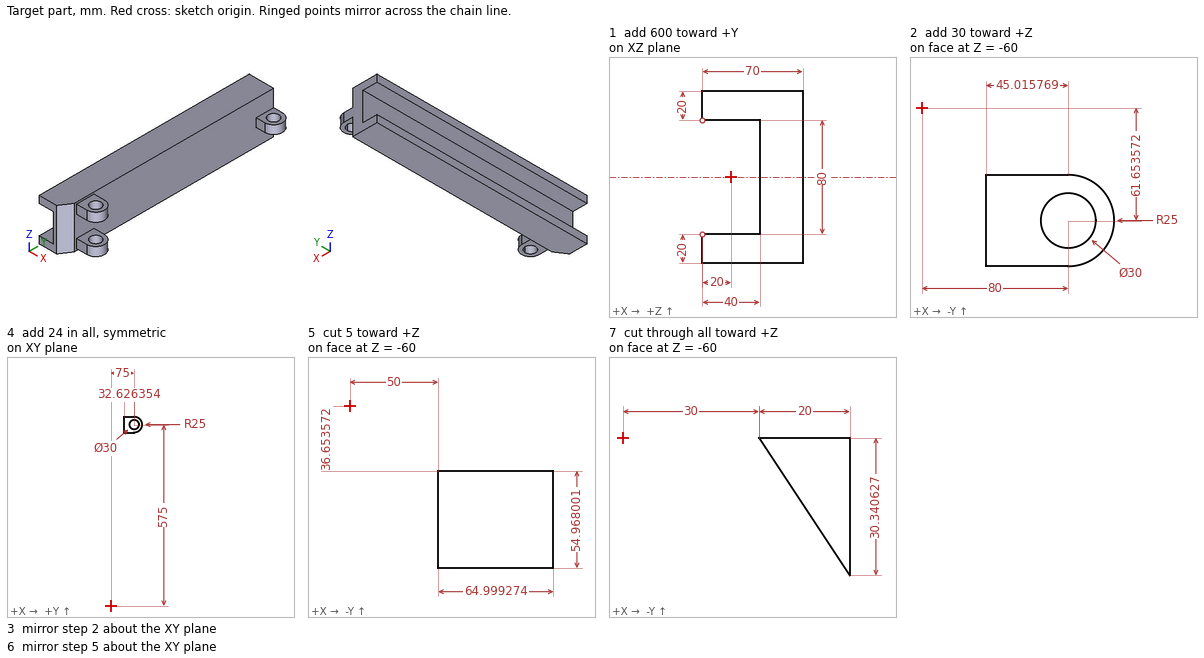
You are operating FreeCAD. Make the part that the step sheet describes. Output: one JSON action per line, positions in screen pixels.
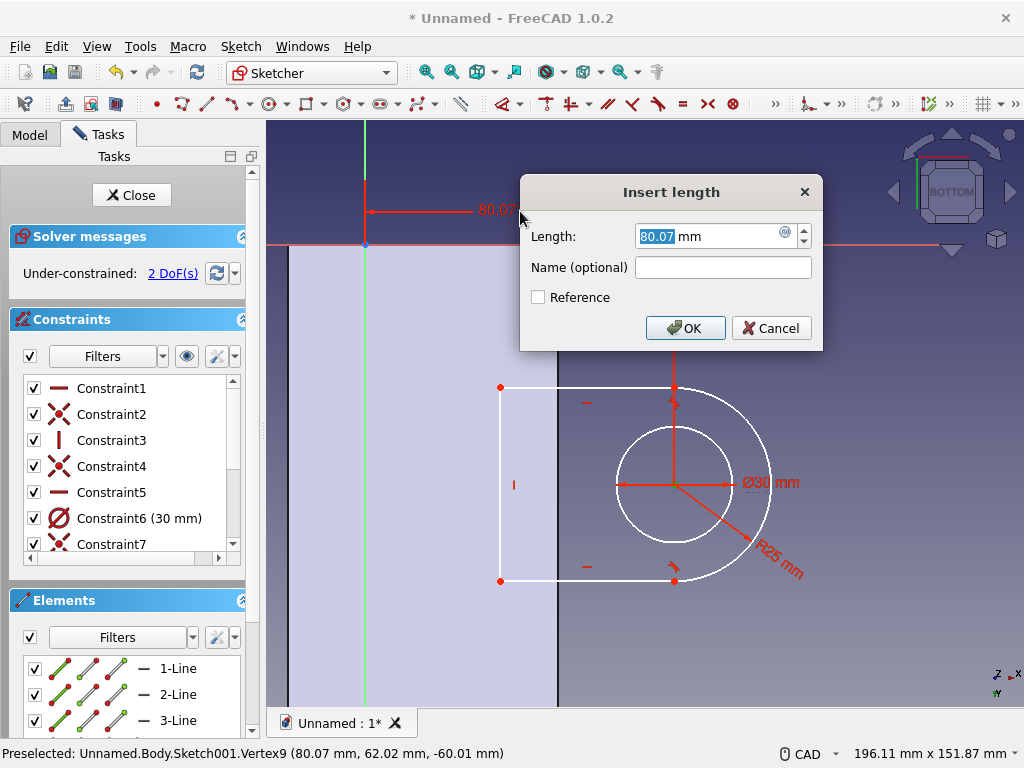
{"action": "type", "text": "80"}
{"action": "key", "text": "Return"}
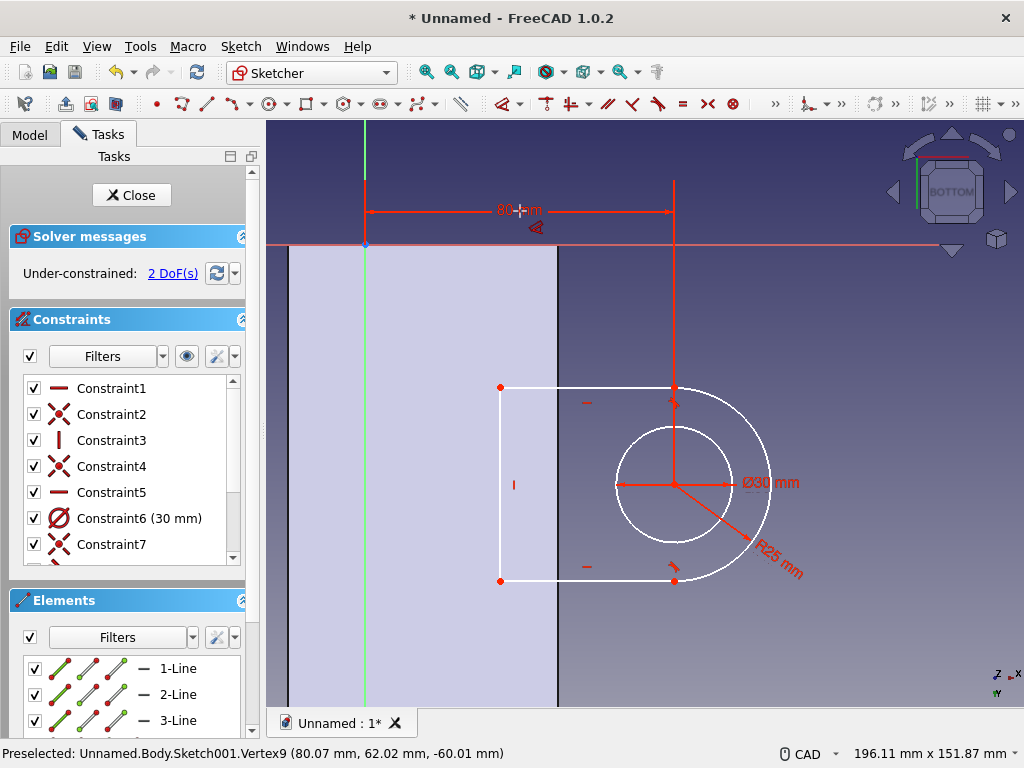
{"action": "left_click", "coordinate": [622, 388]}
{"action": "left_click", "coordinate": [587, 354]}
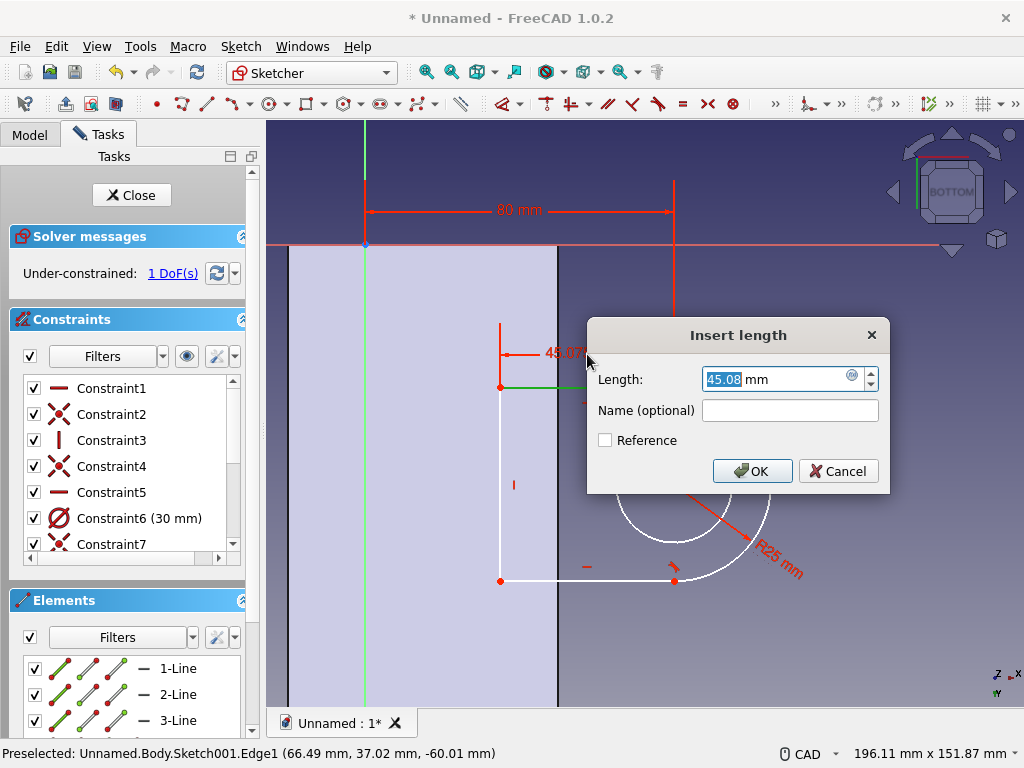
{"action": "type", "text": "45.015769"}
{"action": "key", "text": "Return"}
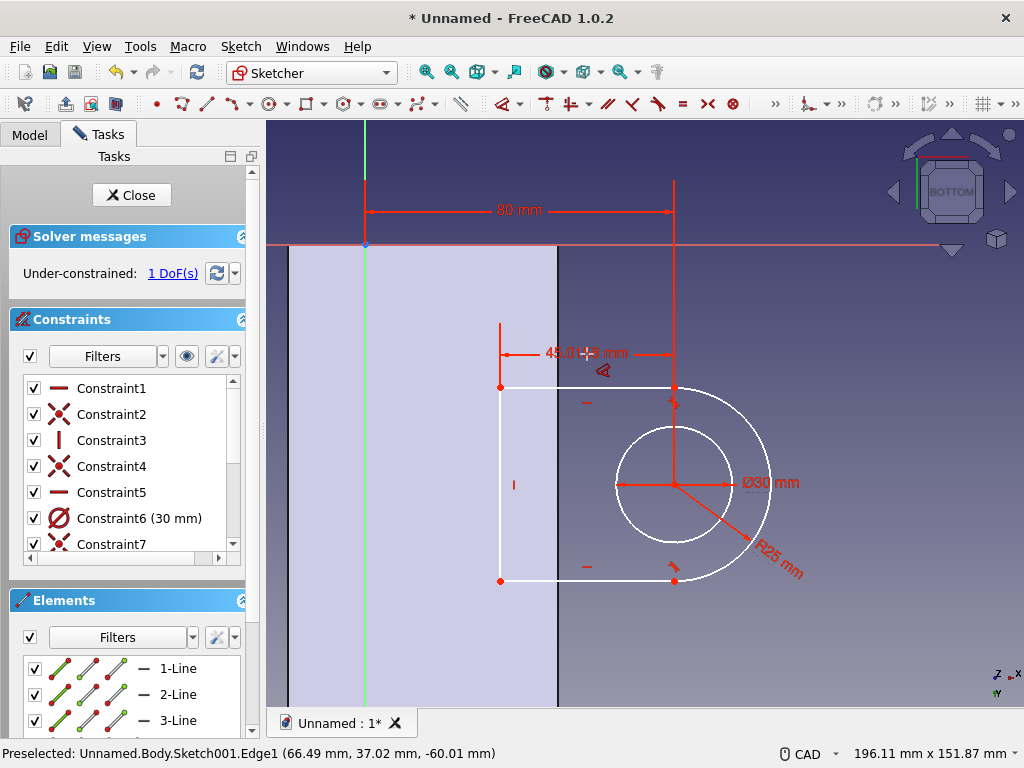
{"action": "left_click", "coordinate": [674, 485]}
{"action": "left_click", "coordinate": [331, 365]}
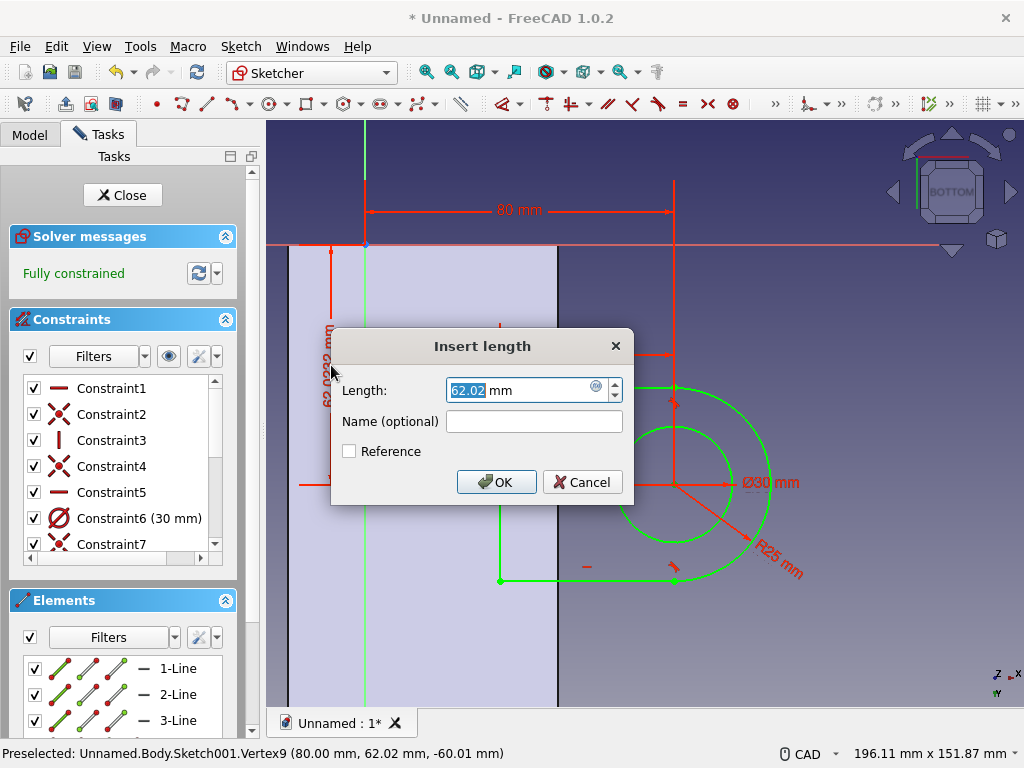
{"action": "type", "text": "61.653572"}
{"action": "key", "text": "Return"}
{"action": "key", "text": "Escape"}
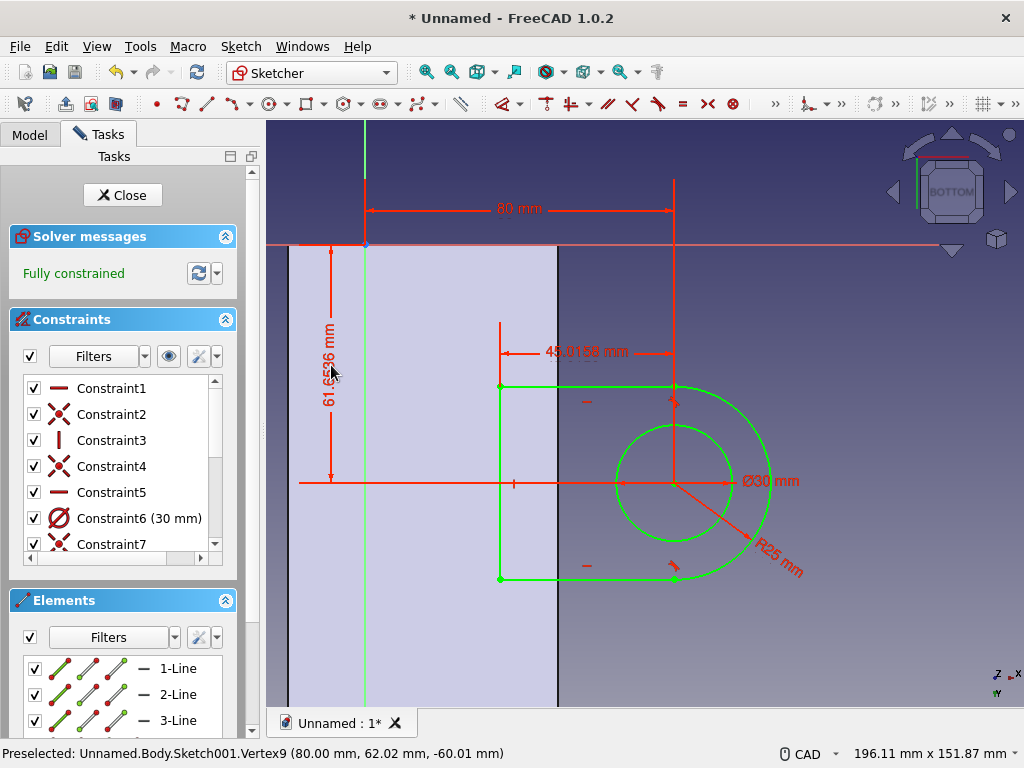
{"action": "left_click", "coordinate": [123, 195]}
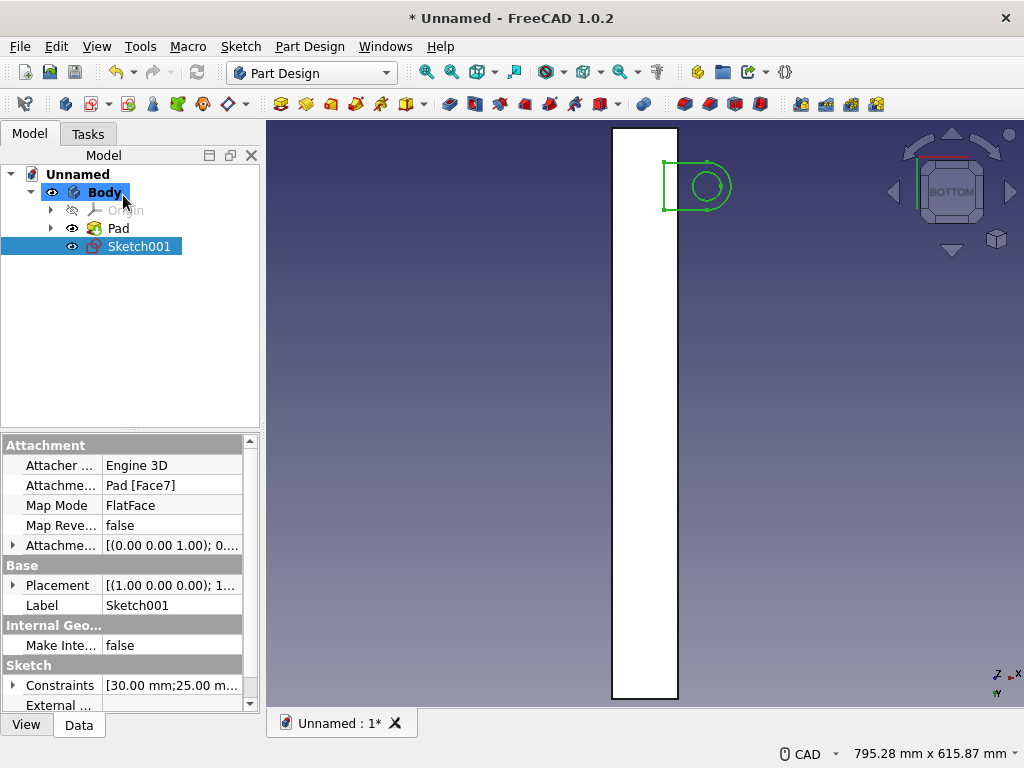
{"action": "left_click", "coordinate": [281, 104]}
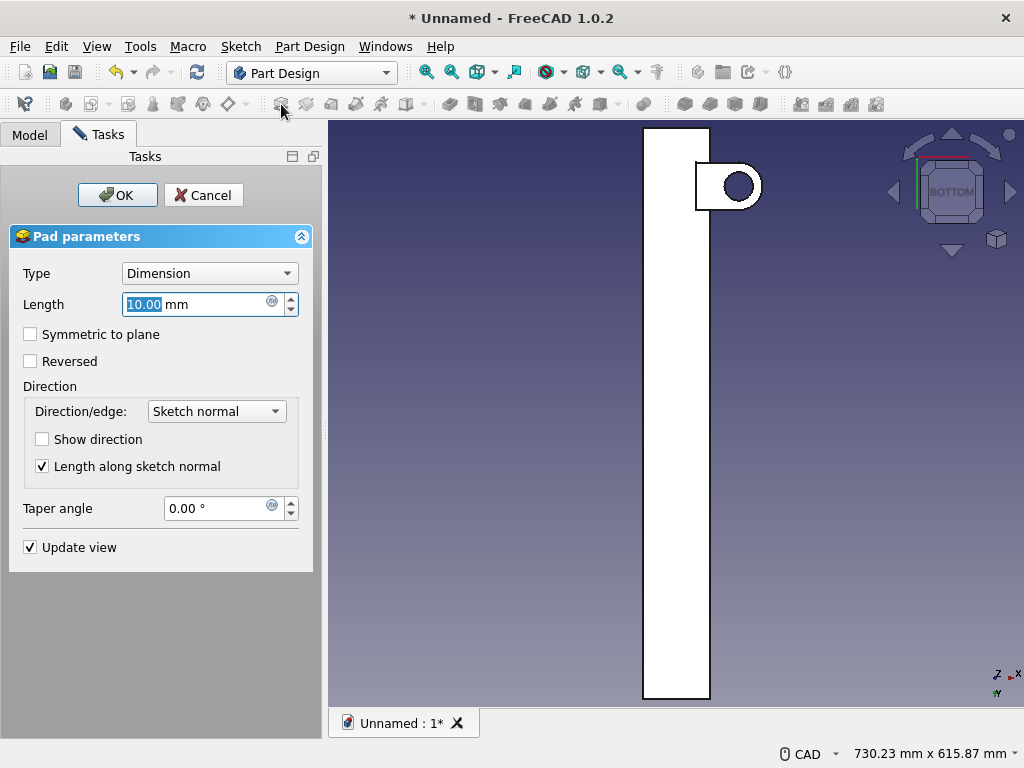
{"action": "type", "text": "30"}
{"action": "key", "text": "Tab"}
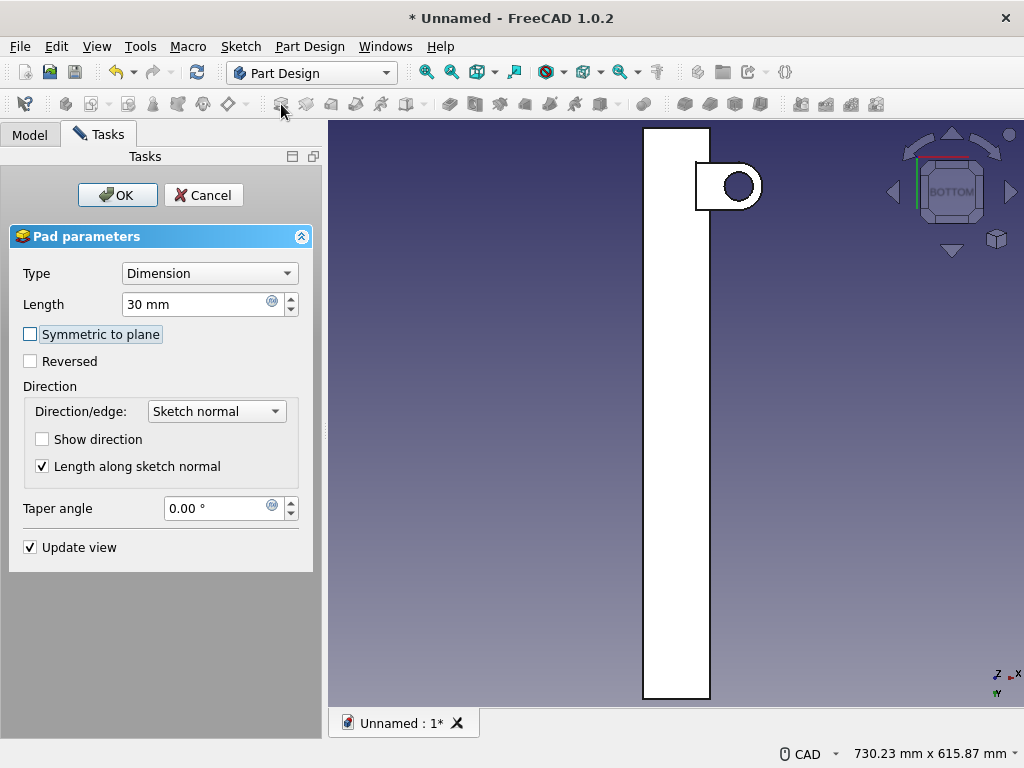
{"action": "left_click", "coordinate": [31, 361]}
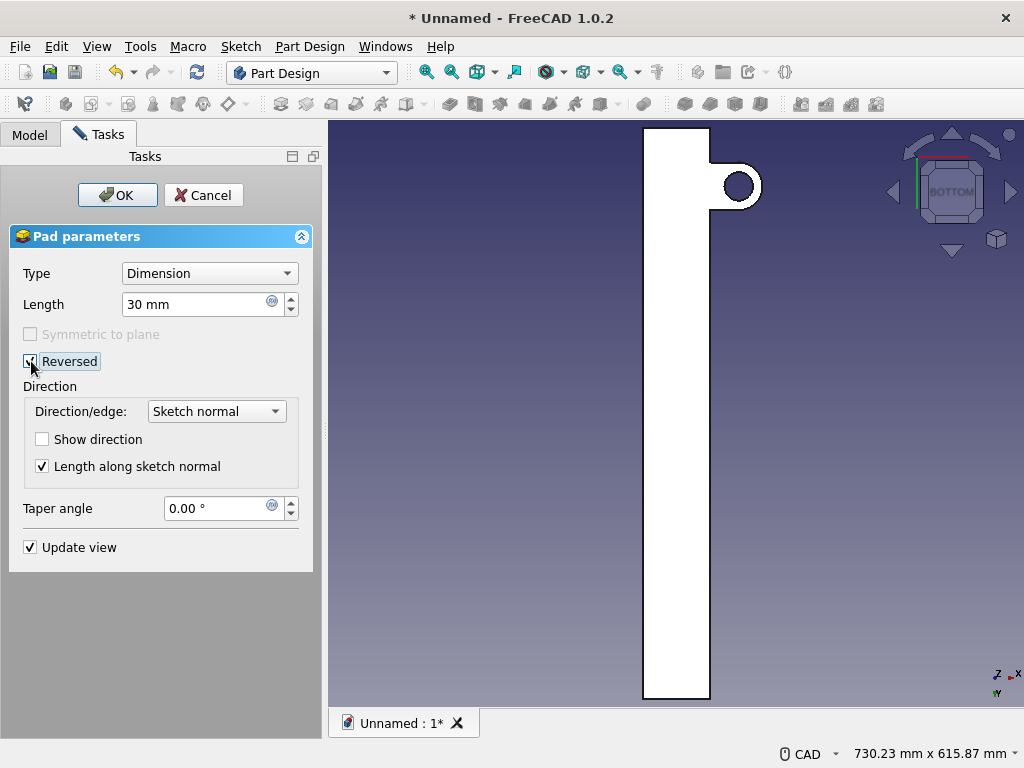
{"action": "left_click", "coordinate": [118, 195]}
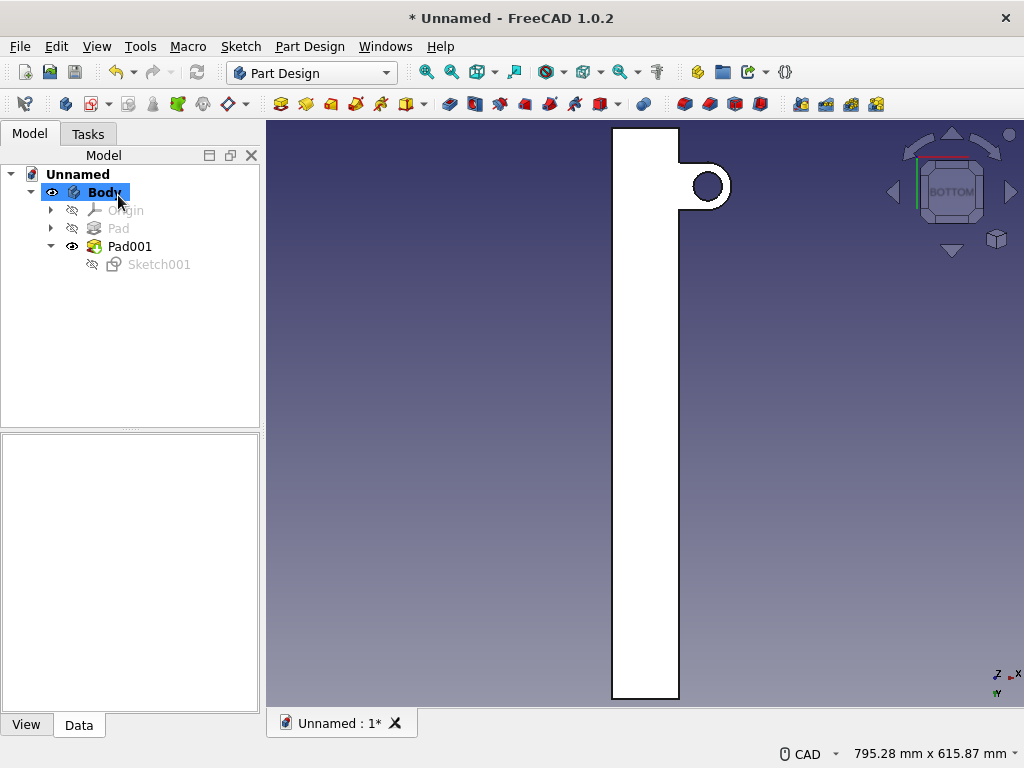
{"action": "left_click", "coordinate": [117, 246]}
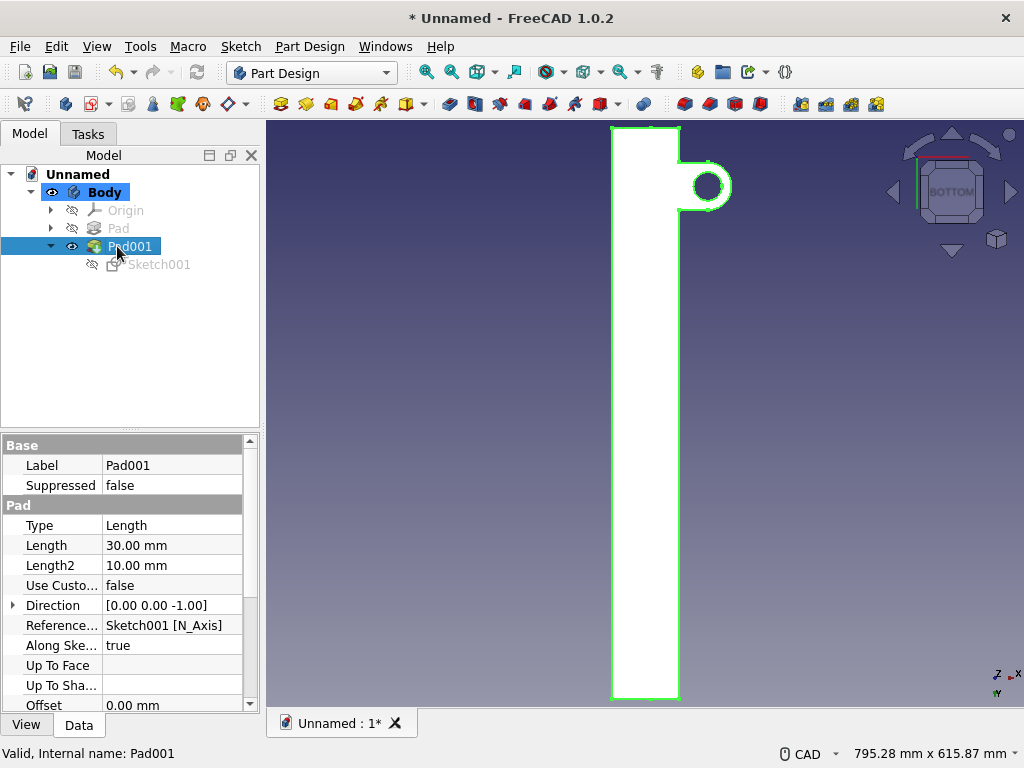
{"action": "left_click", "coordinate": [801, 104]}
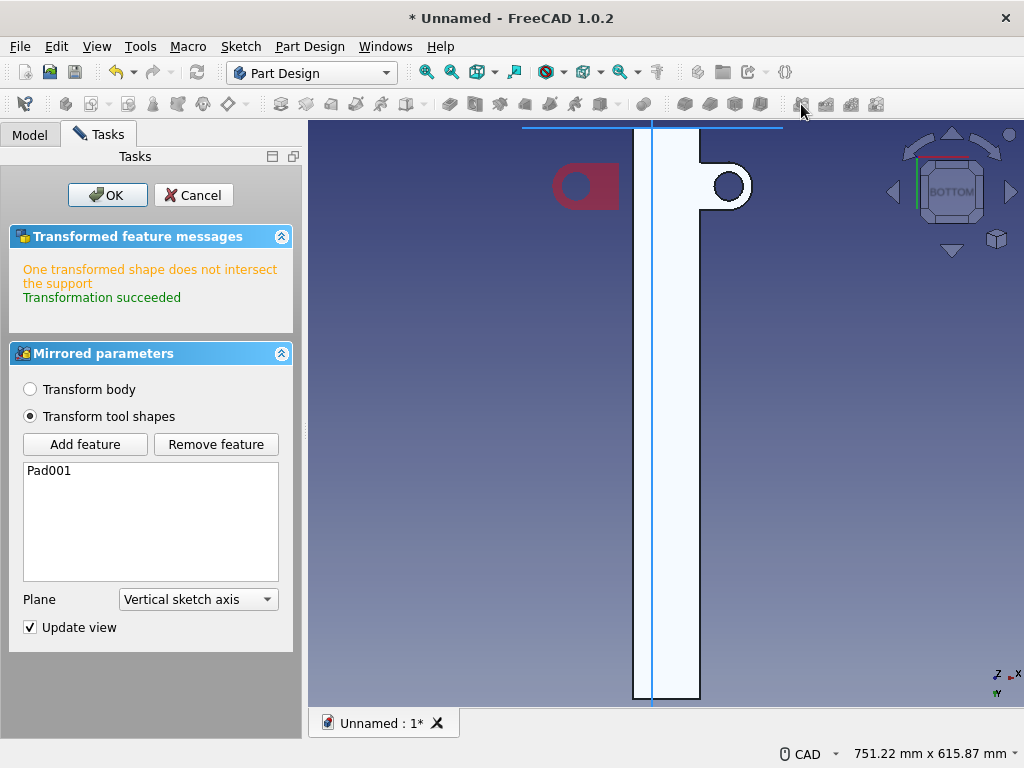
{"action": "left_click", "coordinate": [199, 600]}